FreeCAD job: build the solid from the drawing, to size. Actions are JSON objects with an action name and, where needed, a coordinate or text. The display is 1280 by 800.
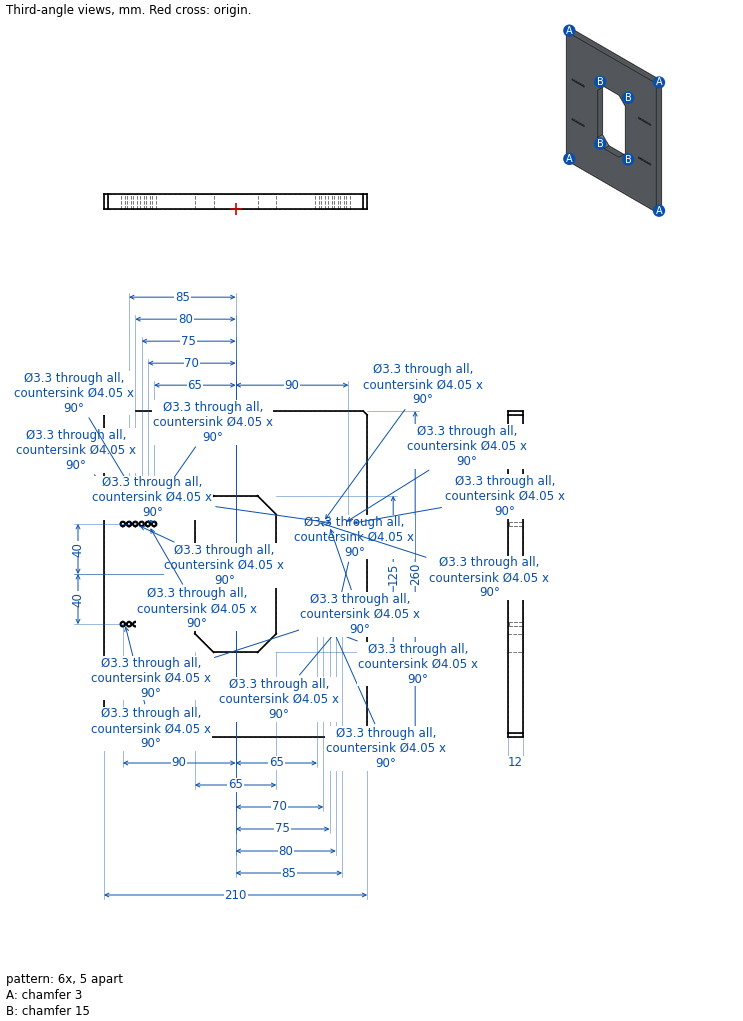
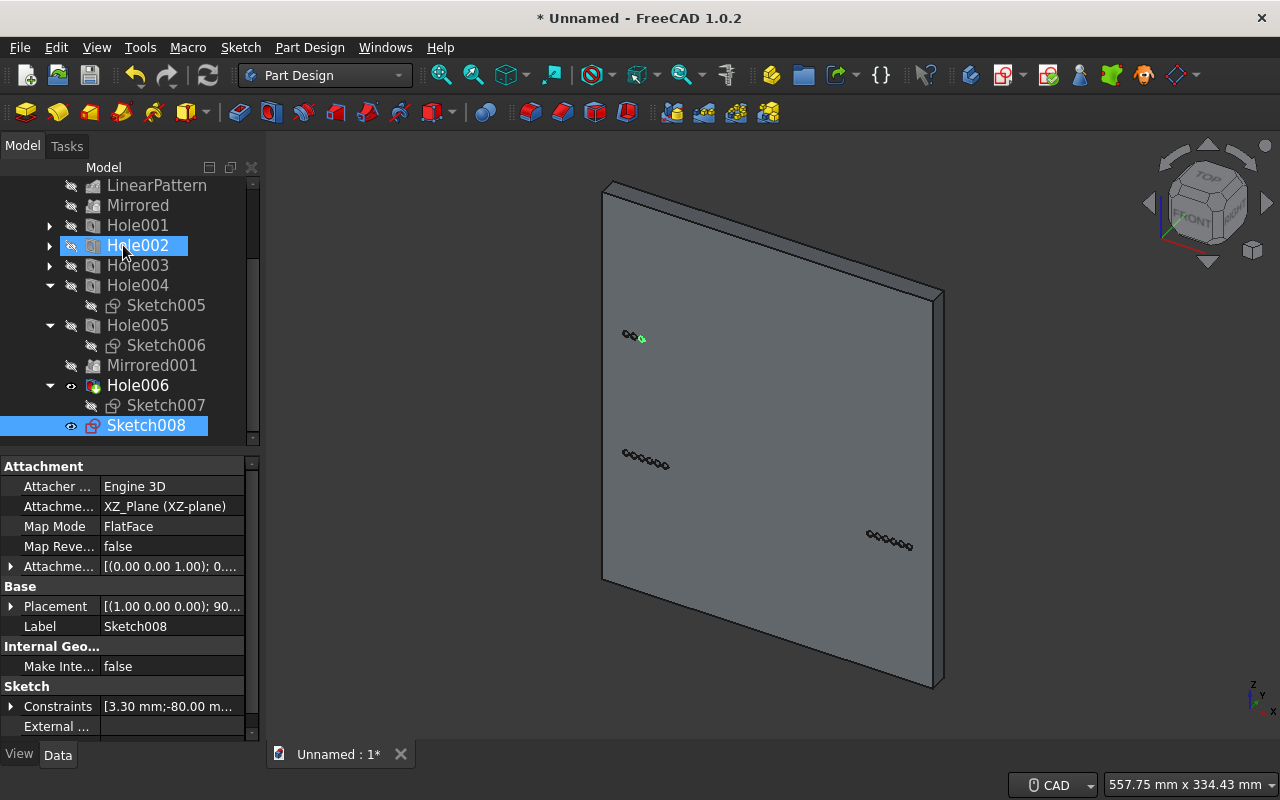
{"action": "left_click", "coordinate": [272, 112]}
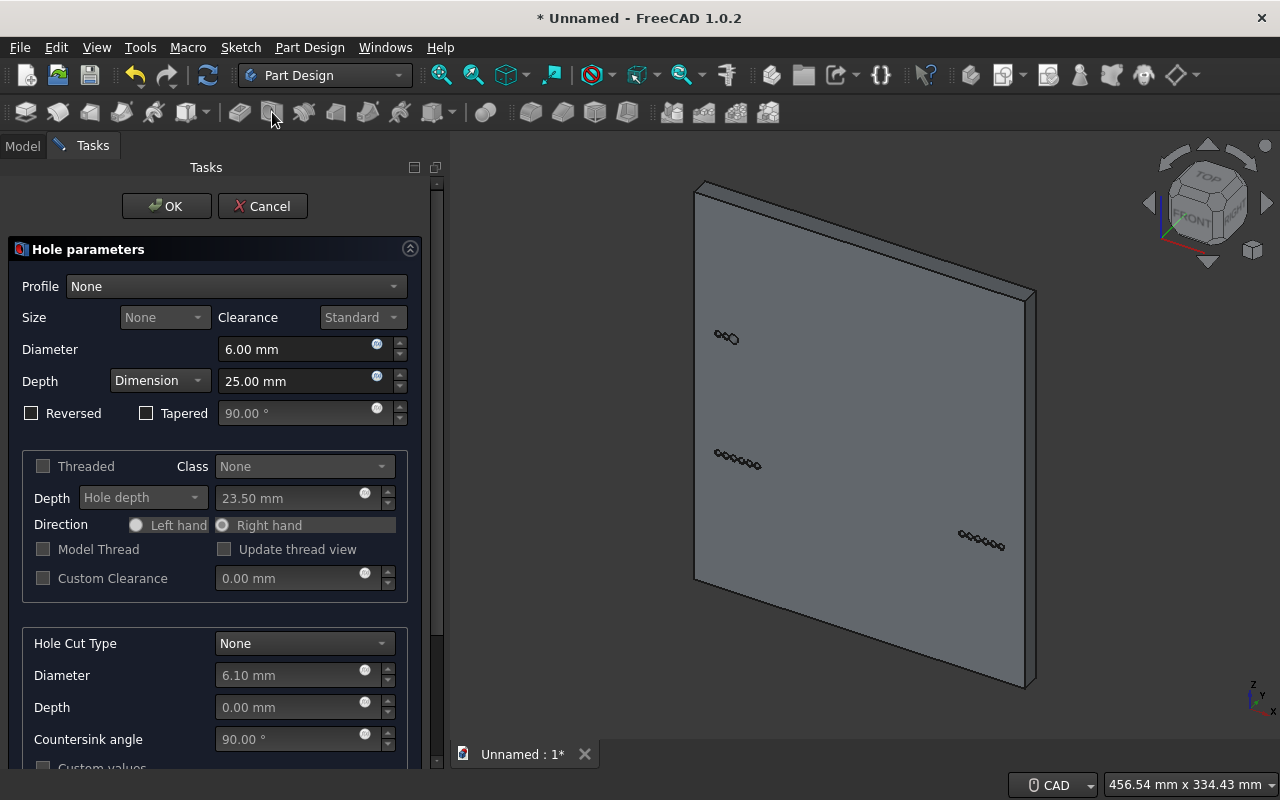
{"action": "triple_click", "coordinate": [305, 349]}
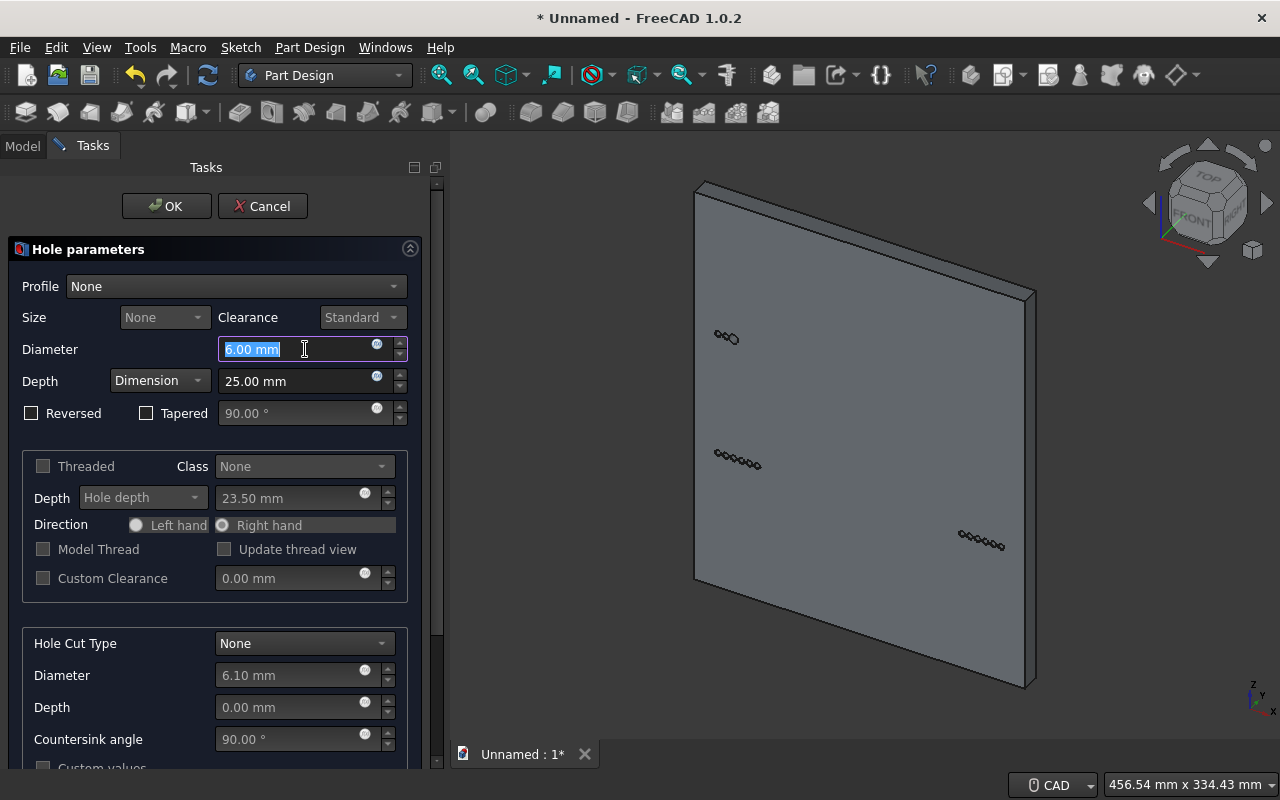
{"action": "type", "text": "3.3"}
{"action": "key", "text": "Tab"}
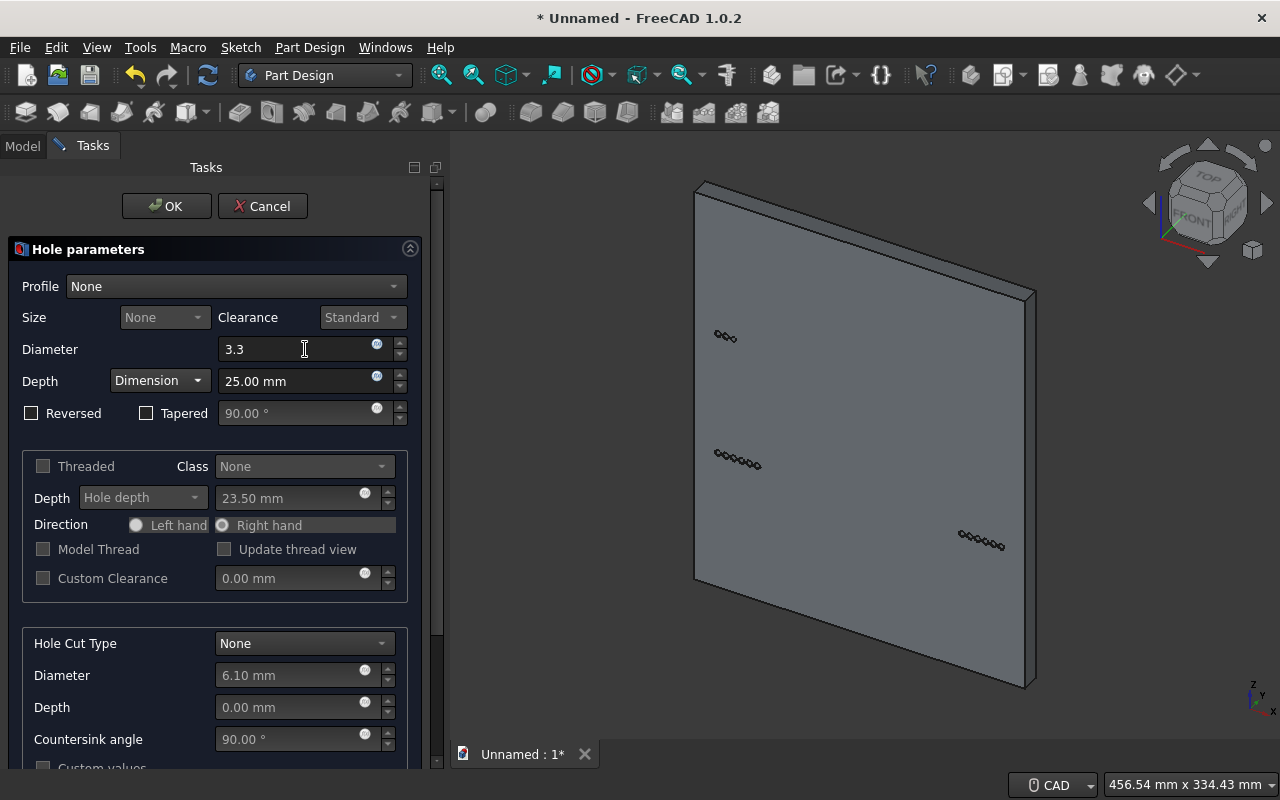
{"action": "left_click", "coordinate": [161, 380]}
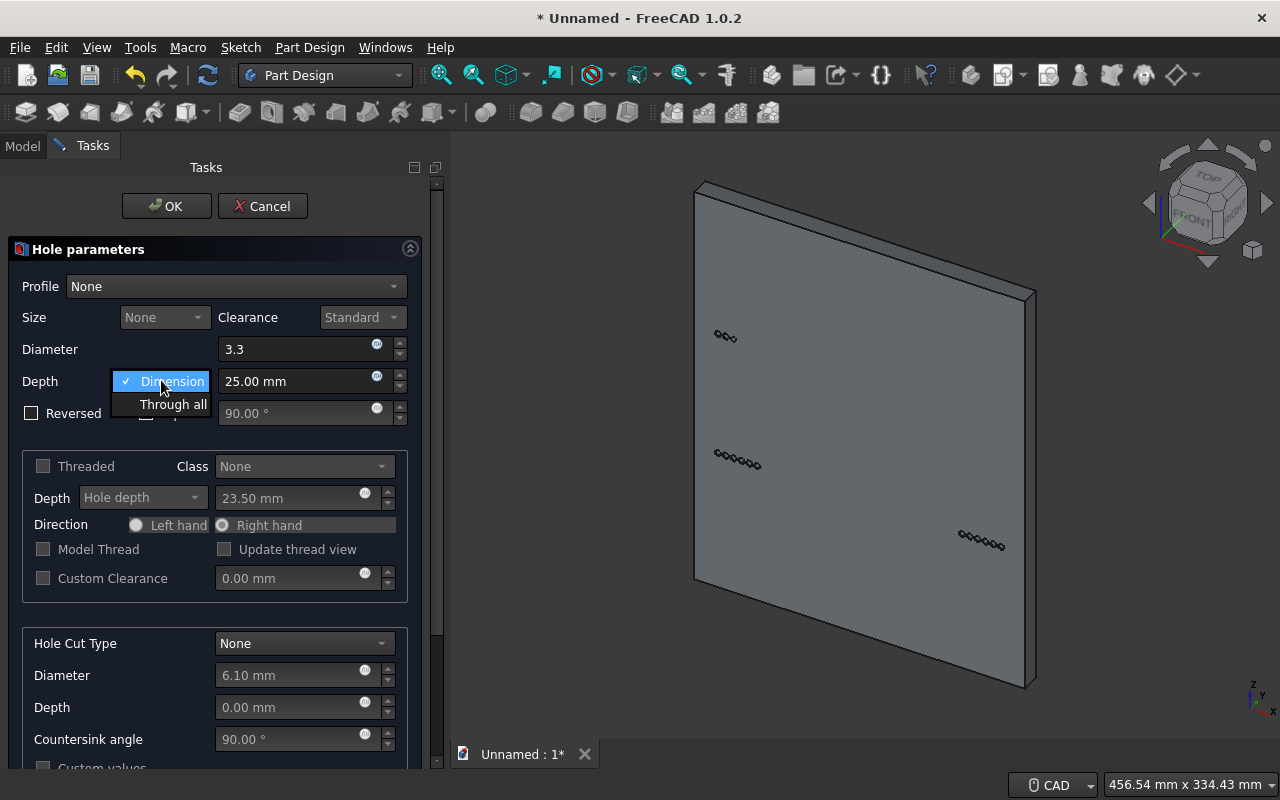
{"action": "left_click", "coordinate": [160, 404]}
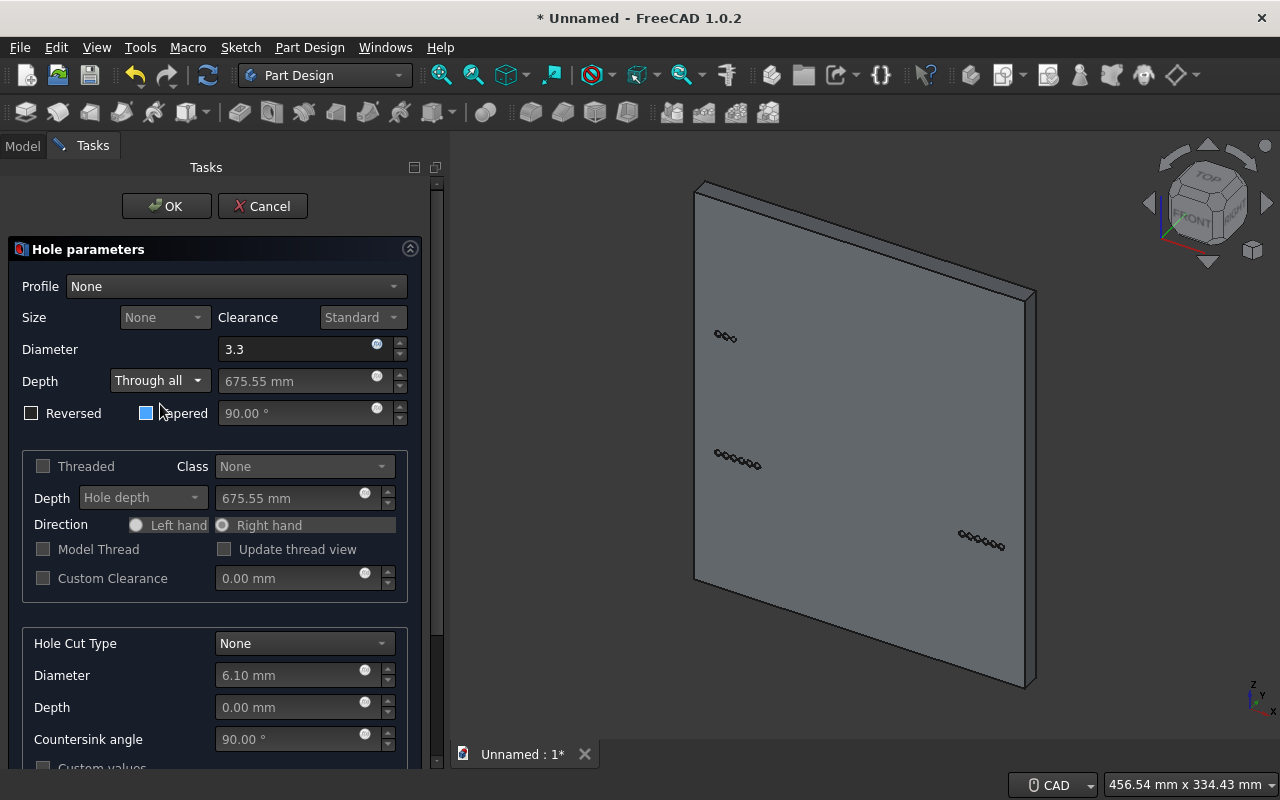
{"action": "left_click", "coordinate": [306, 644]}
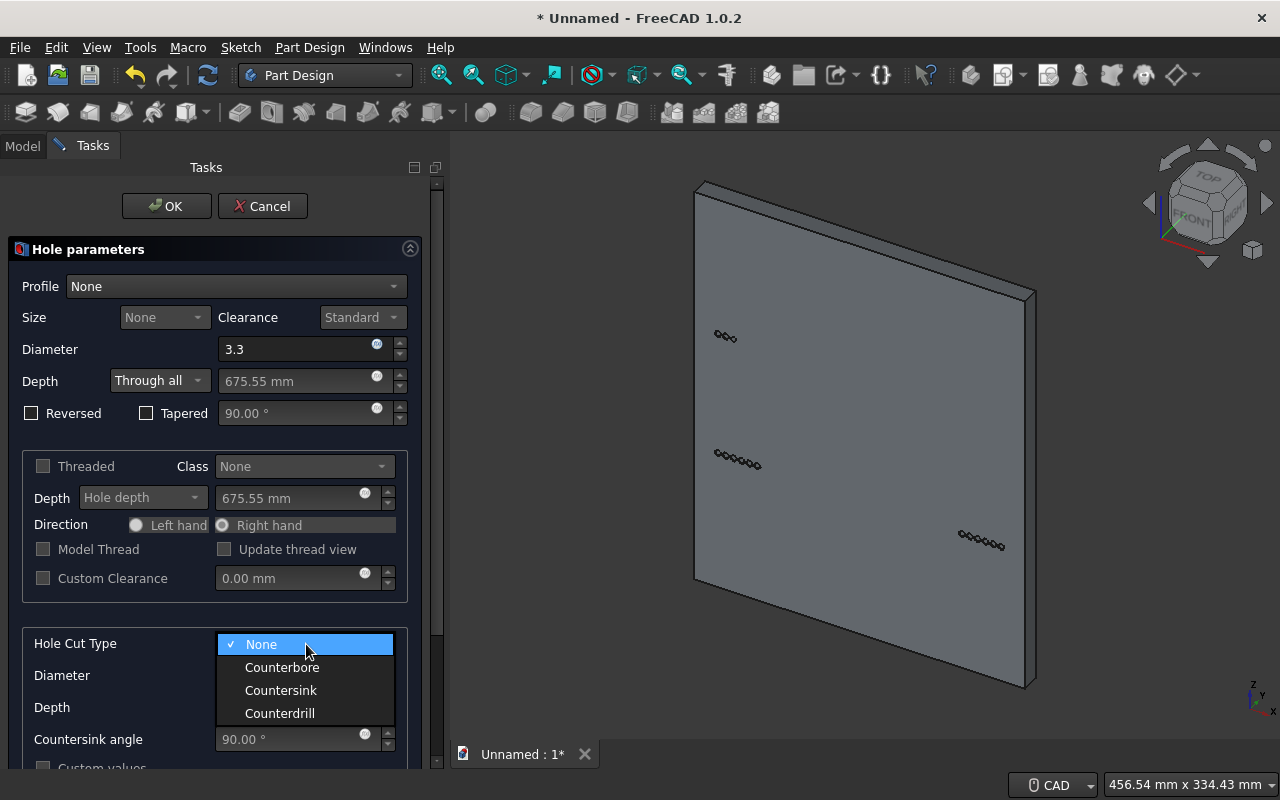
{"action": "left_click", "coordinate": [304, 690]}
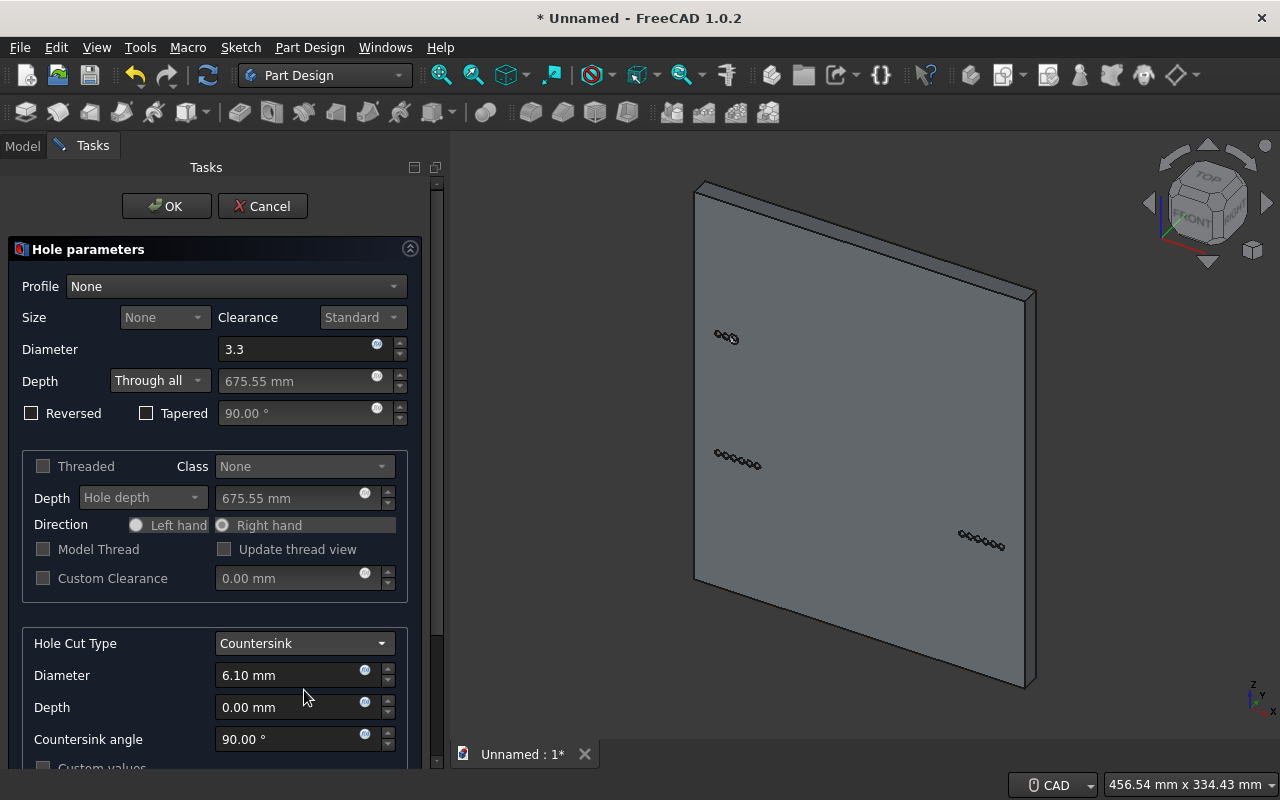
{"action": "triple_click", "coordinate": [298, 675]}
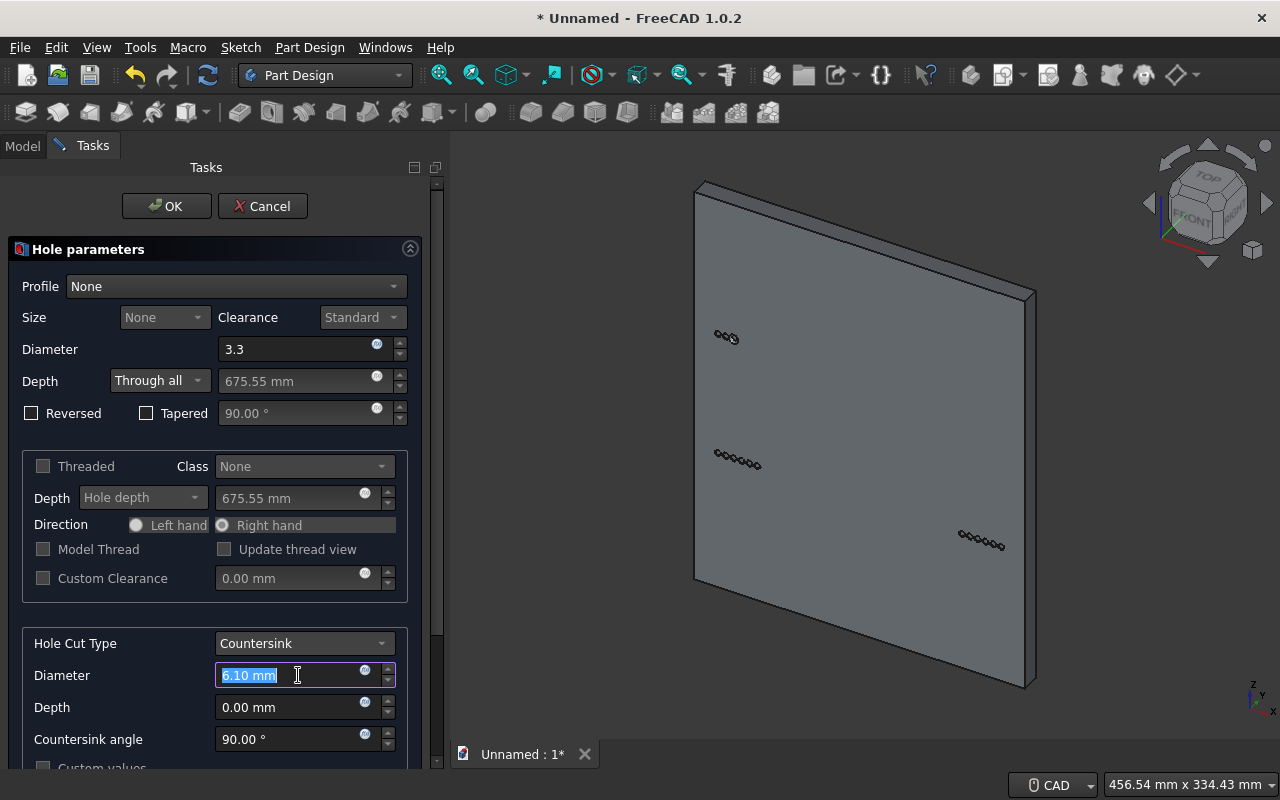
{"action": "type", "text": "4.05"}
{"action": "key", "text": "Tab"}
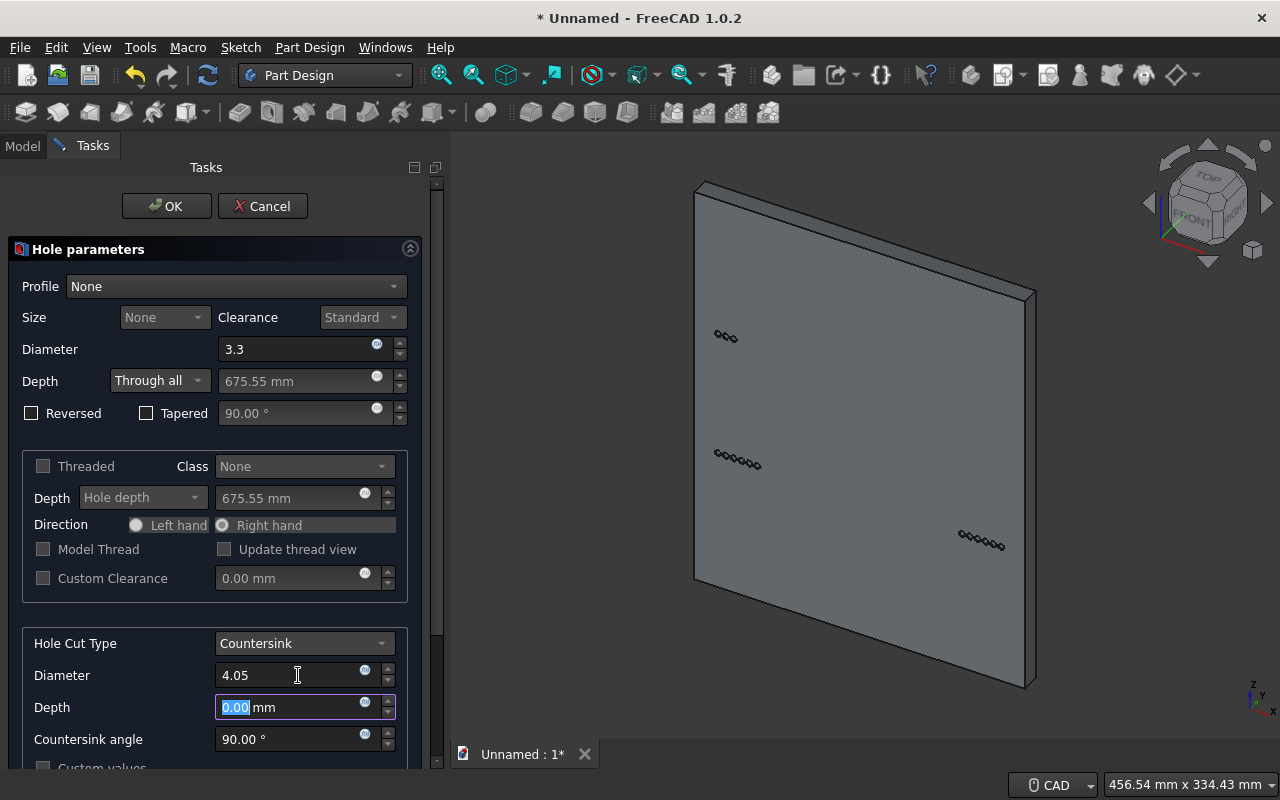
{"action": "left_click", "coordinate": [167, 206]}